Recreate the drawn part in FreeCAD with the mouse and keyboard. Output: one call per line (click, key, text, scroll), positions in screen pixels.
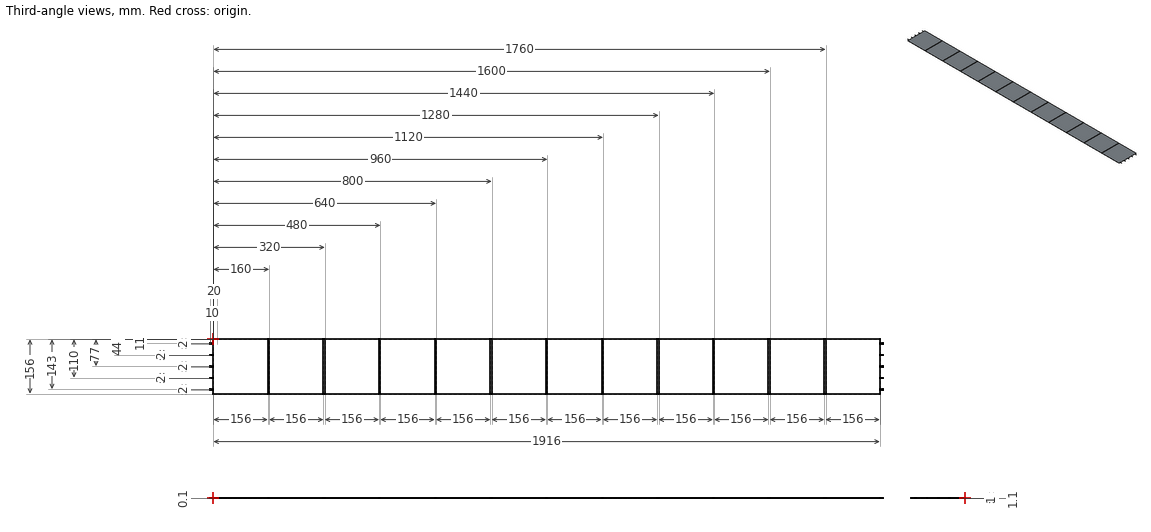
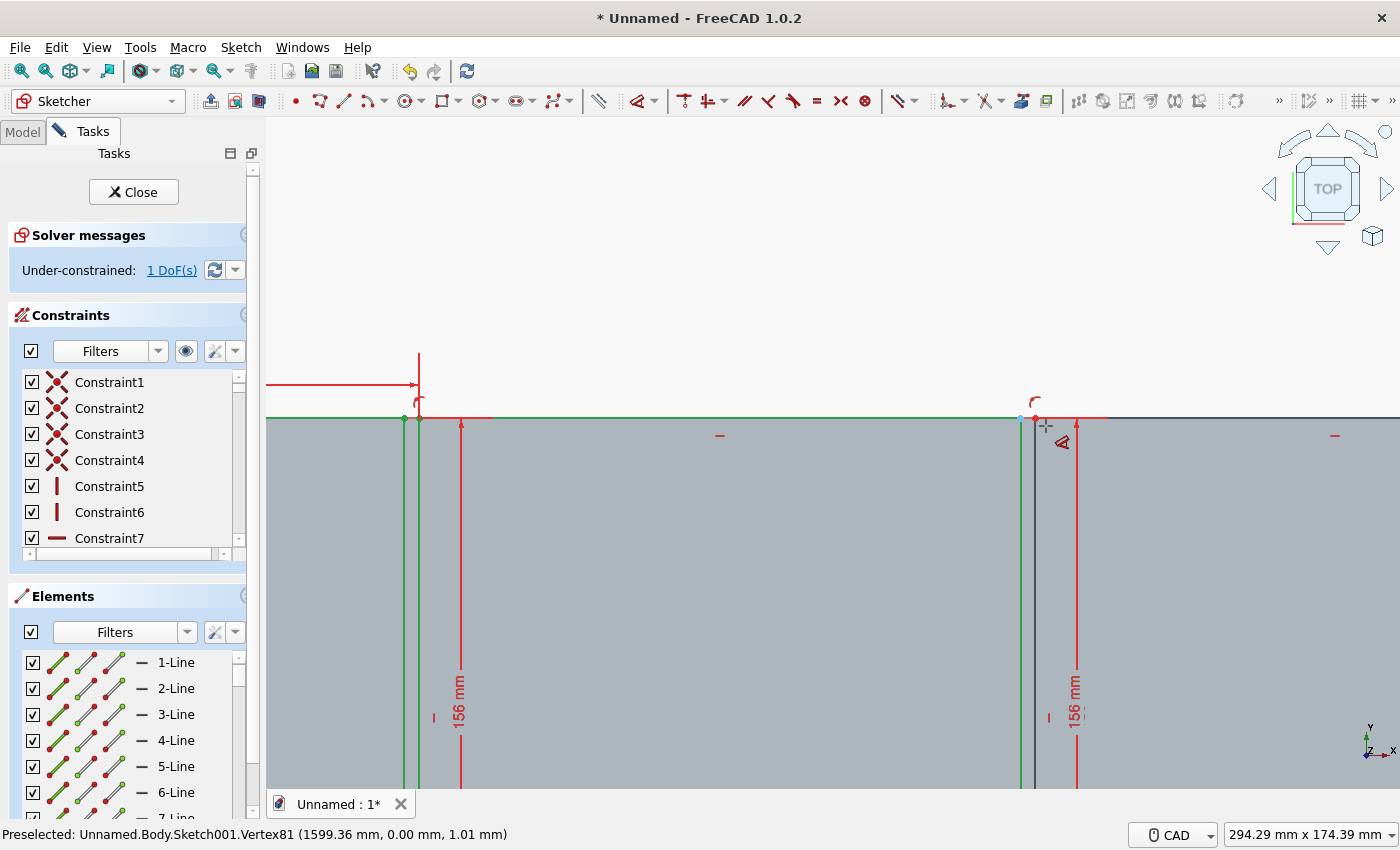
click(1035, 418)
click(665, 384)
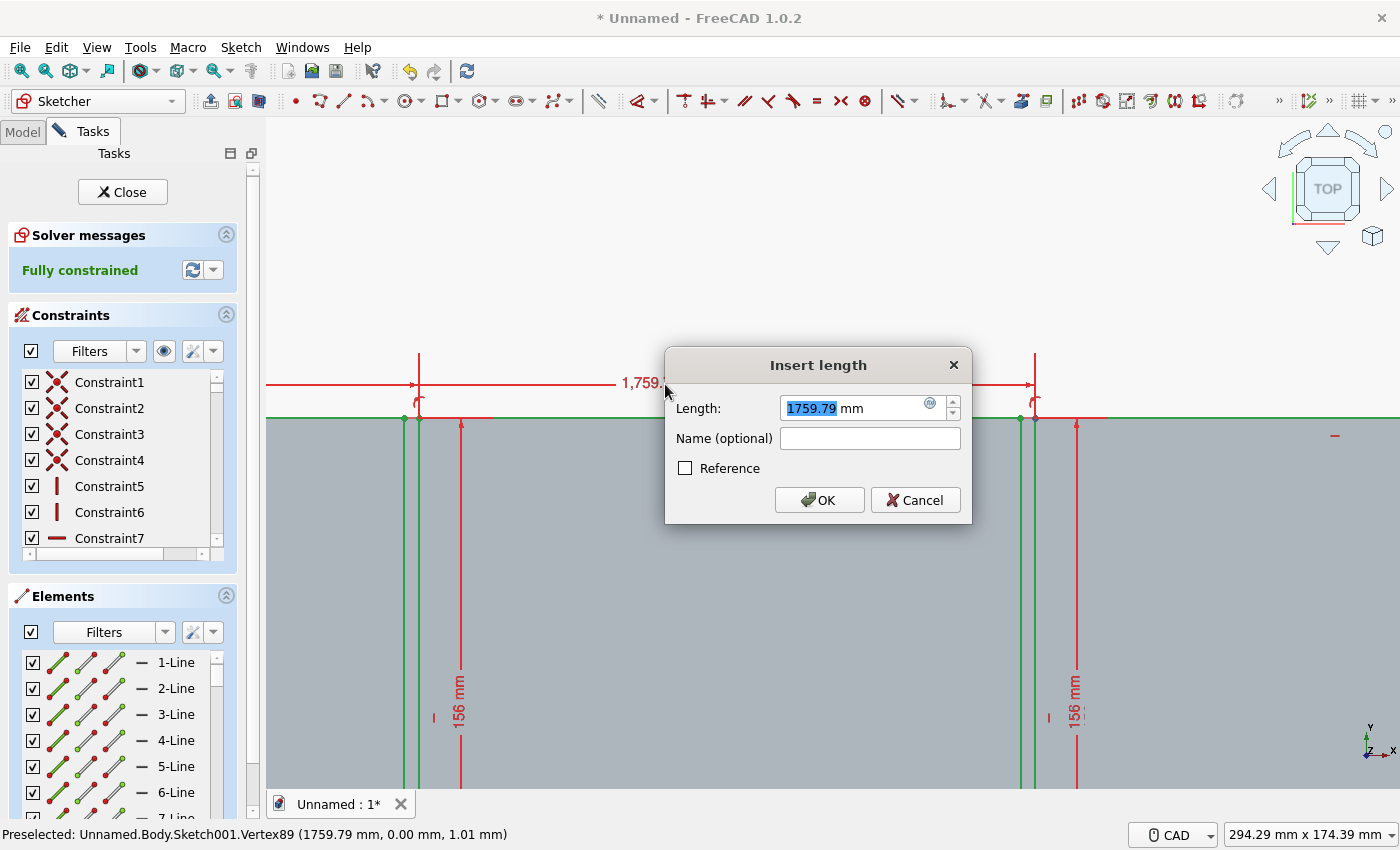
text(1760)
key(Return)
key(Escape)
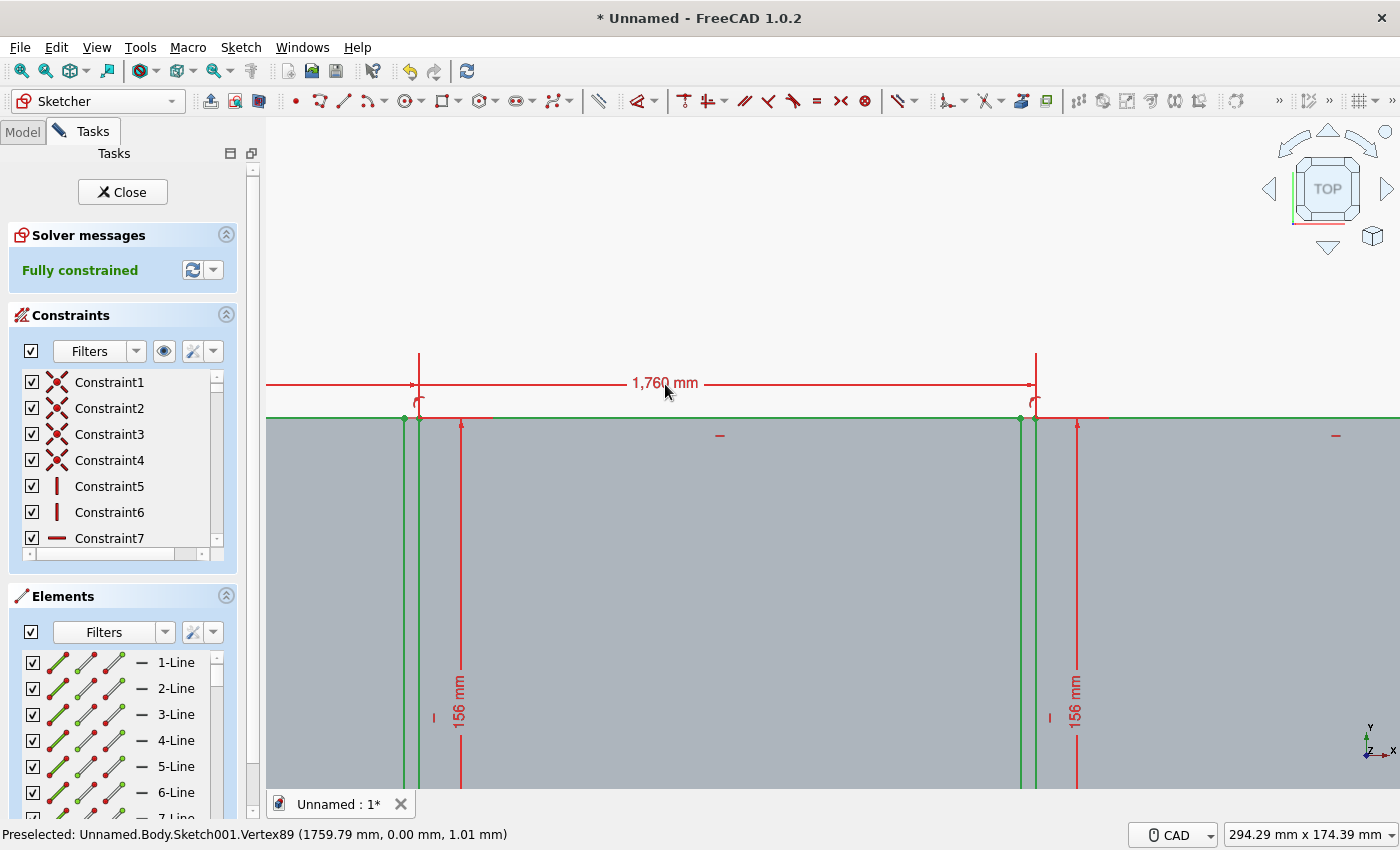
click(123, 192)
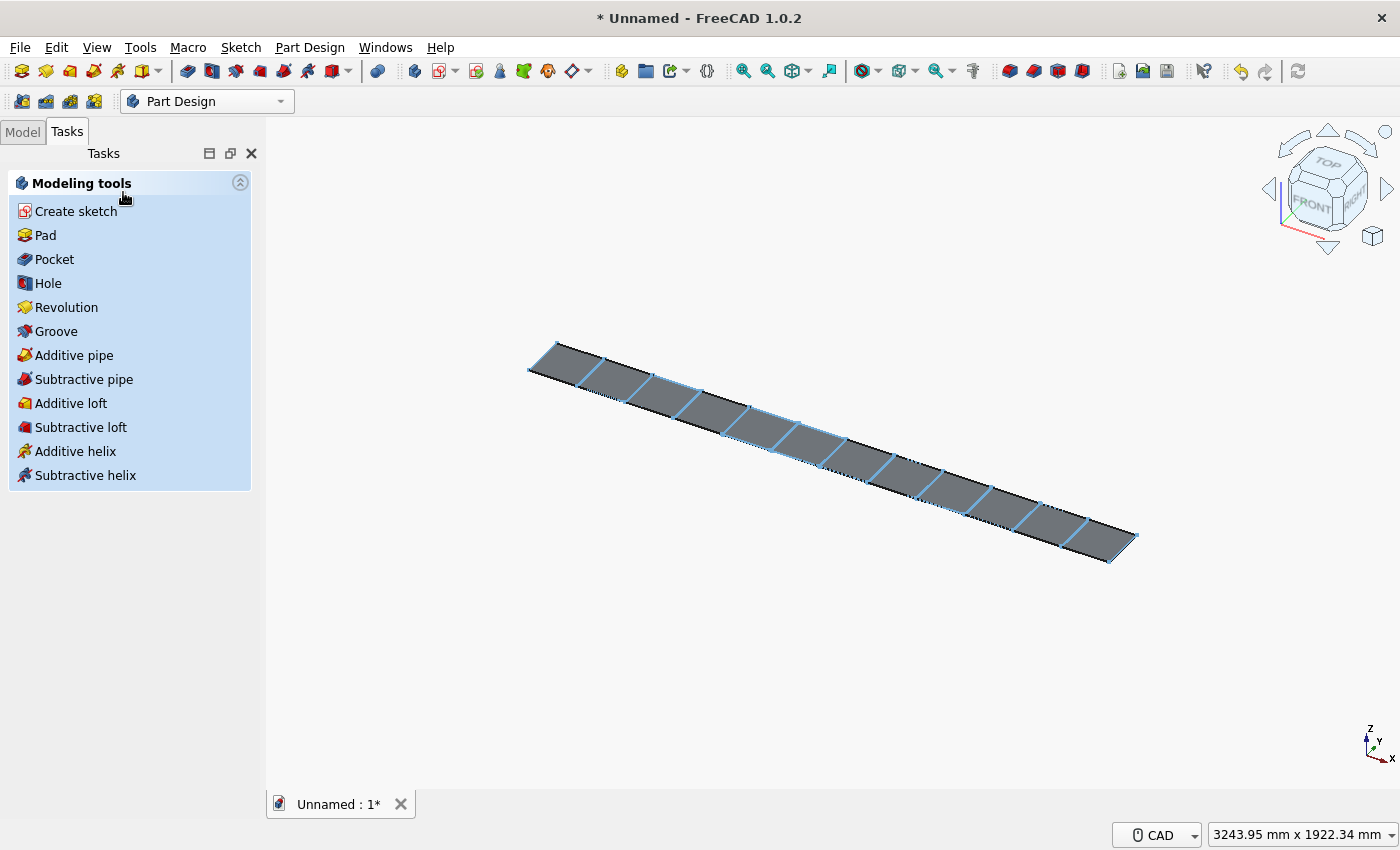
click(22, 72)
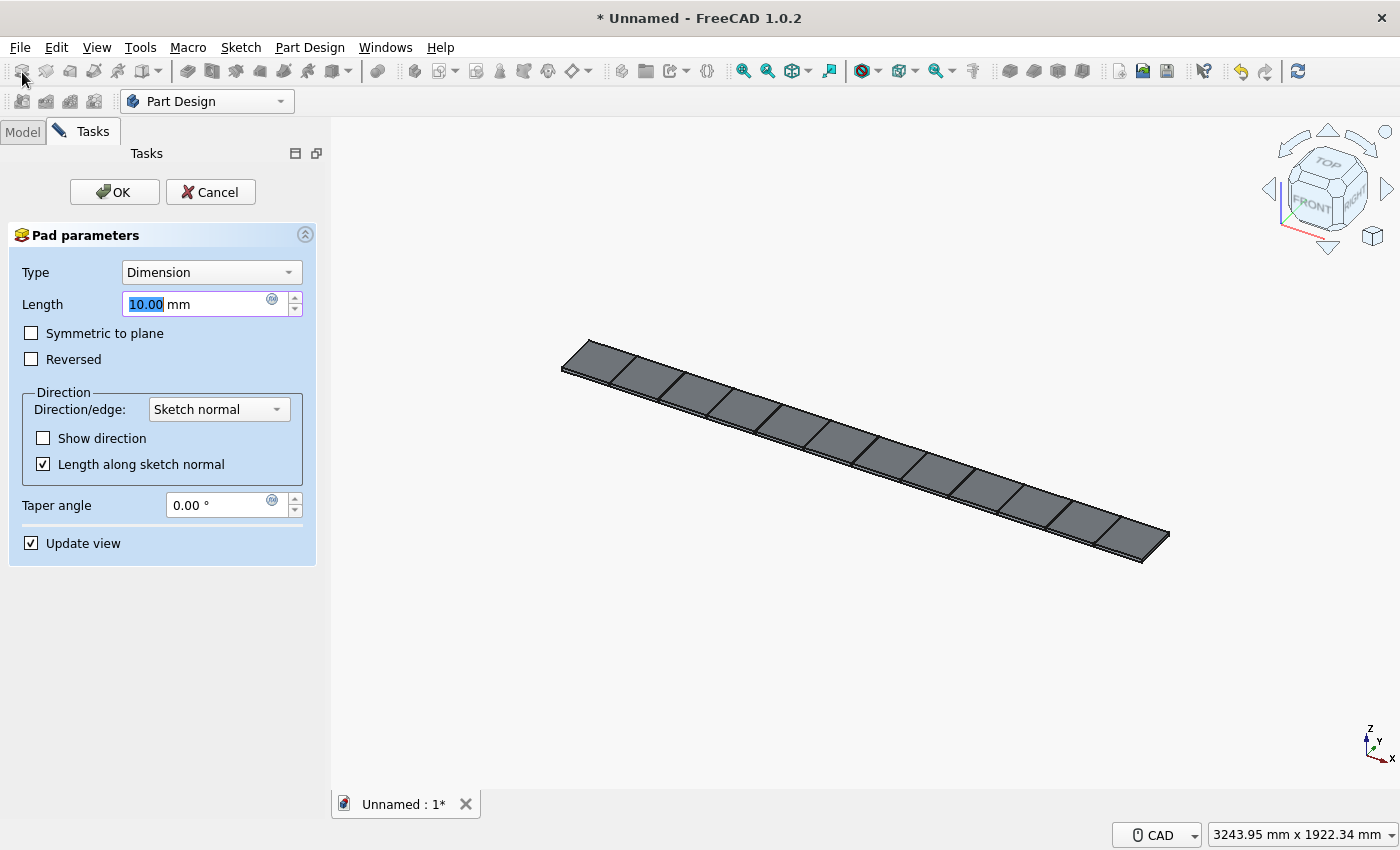
text(0.1)
key(Tab)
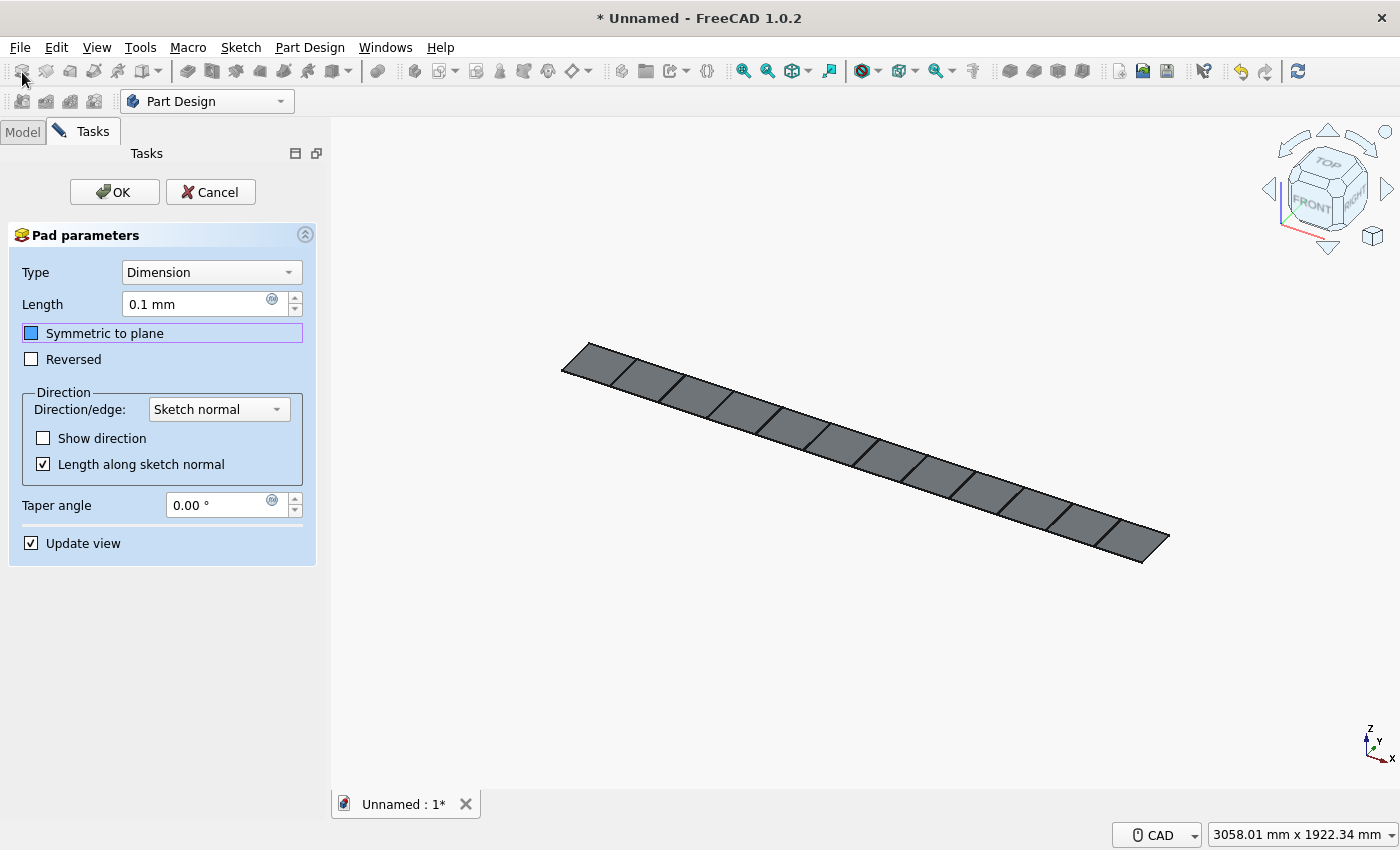
click(115, 192)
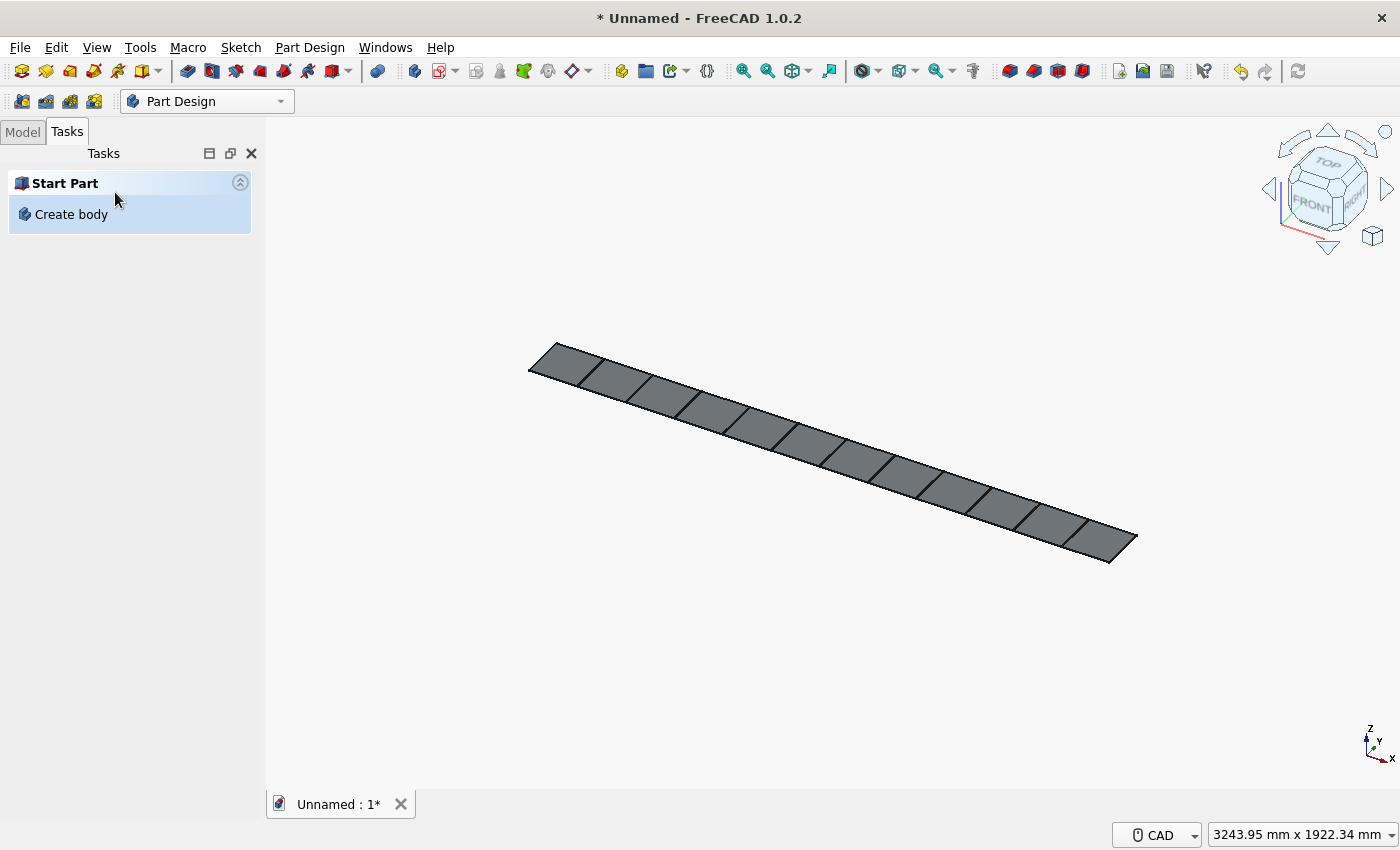
click(663, 396)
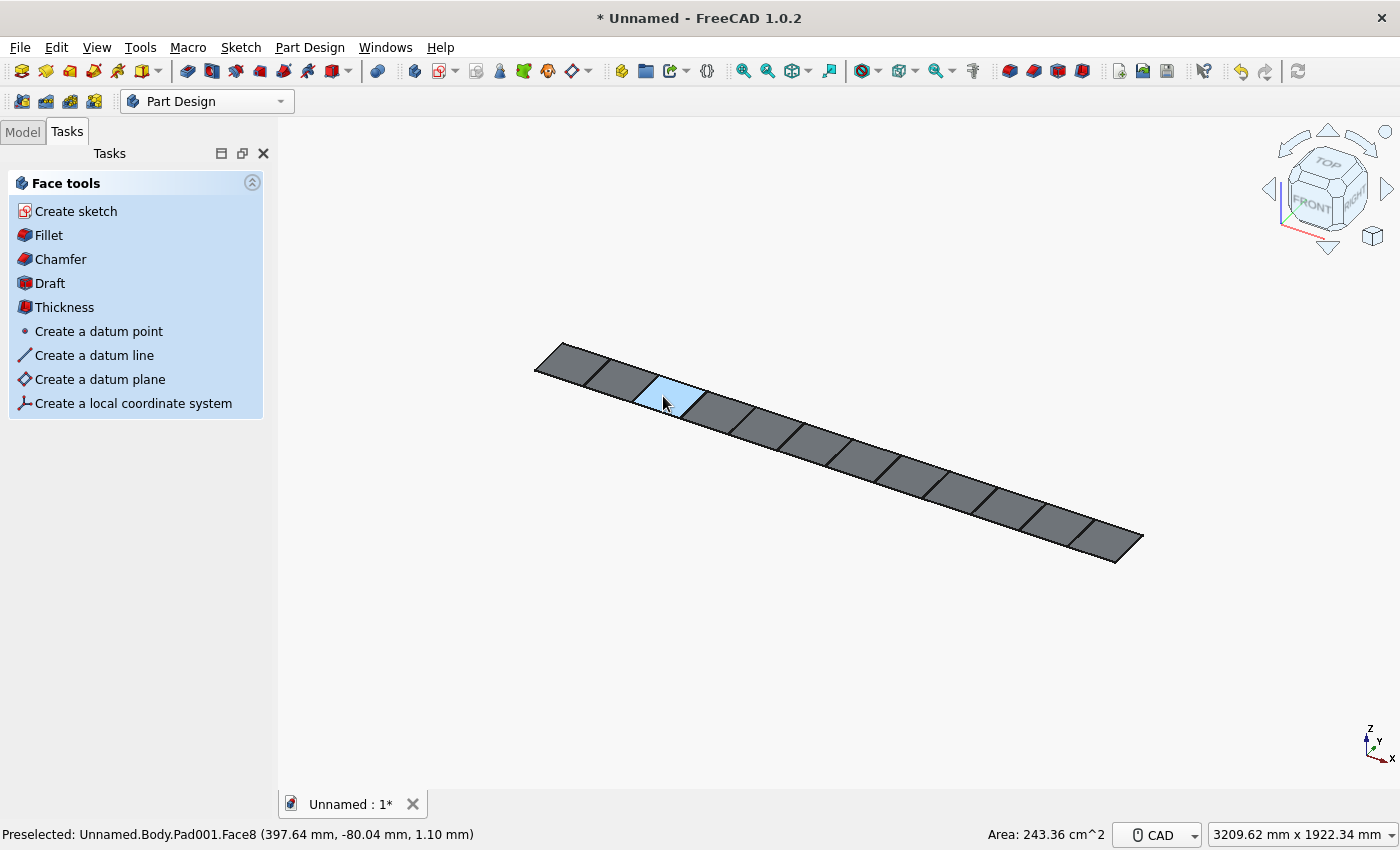
click(440, 72)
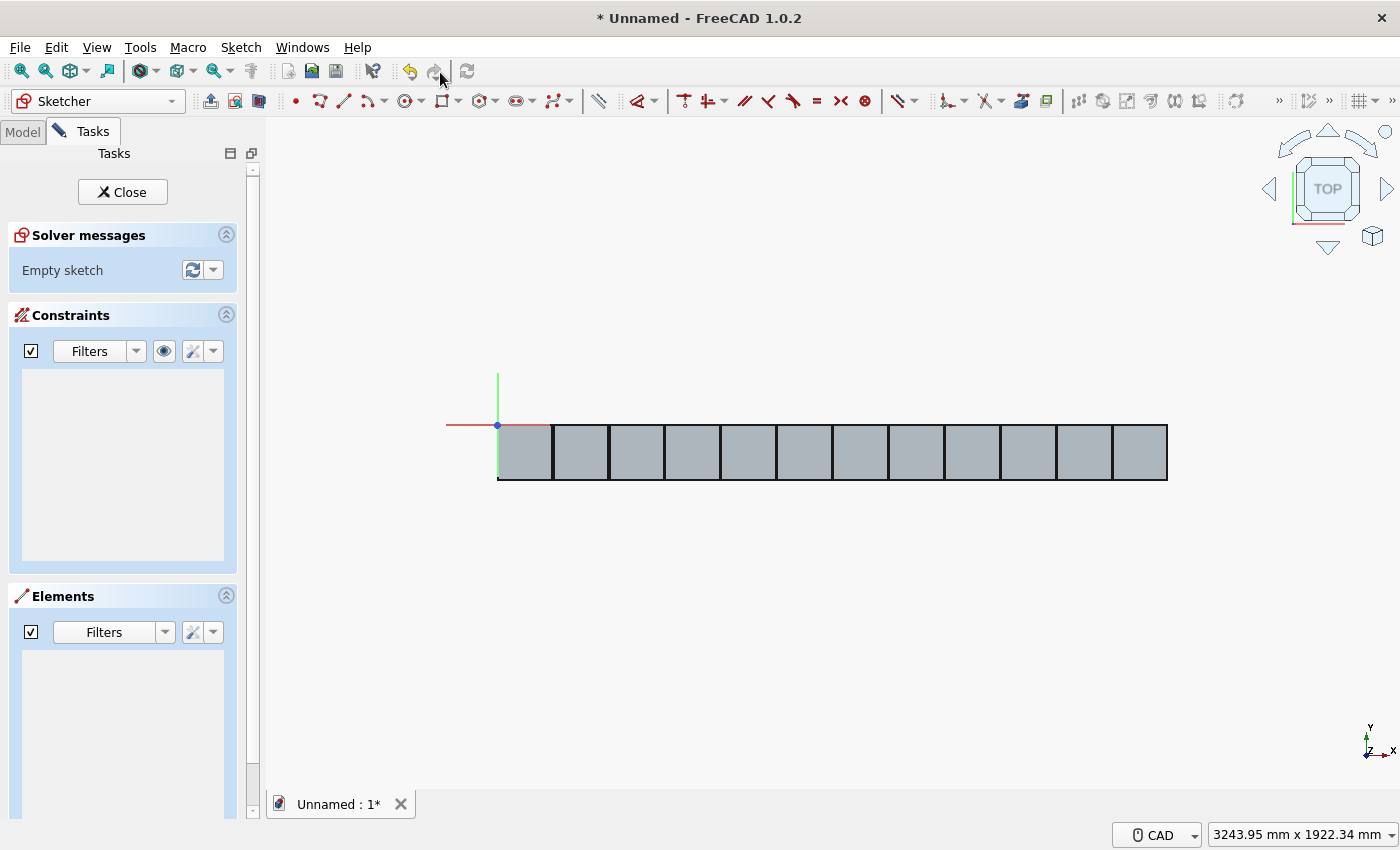
scroll(464, 450, up, 11)